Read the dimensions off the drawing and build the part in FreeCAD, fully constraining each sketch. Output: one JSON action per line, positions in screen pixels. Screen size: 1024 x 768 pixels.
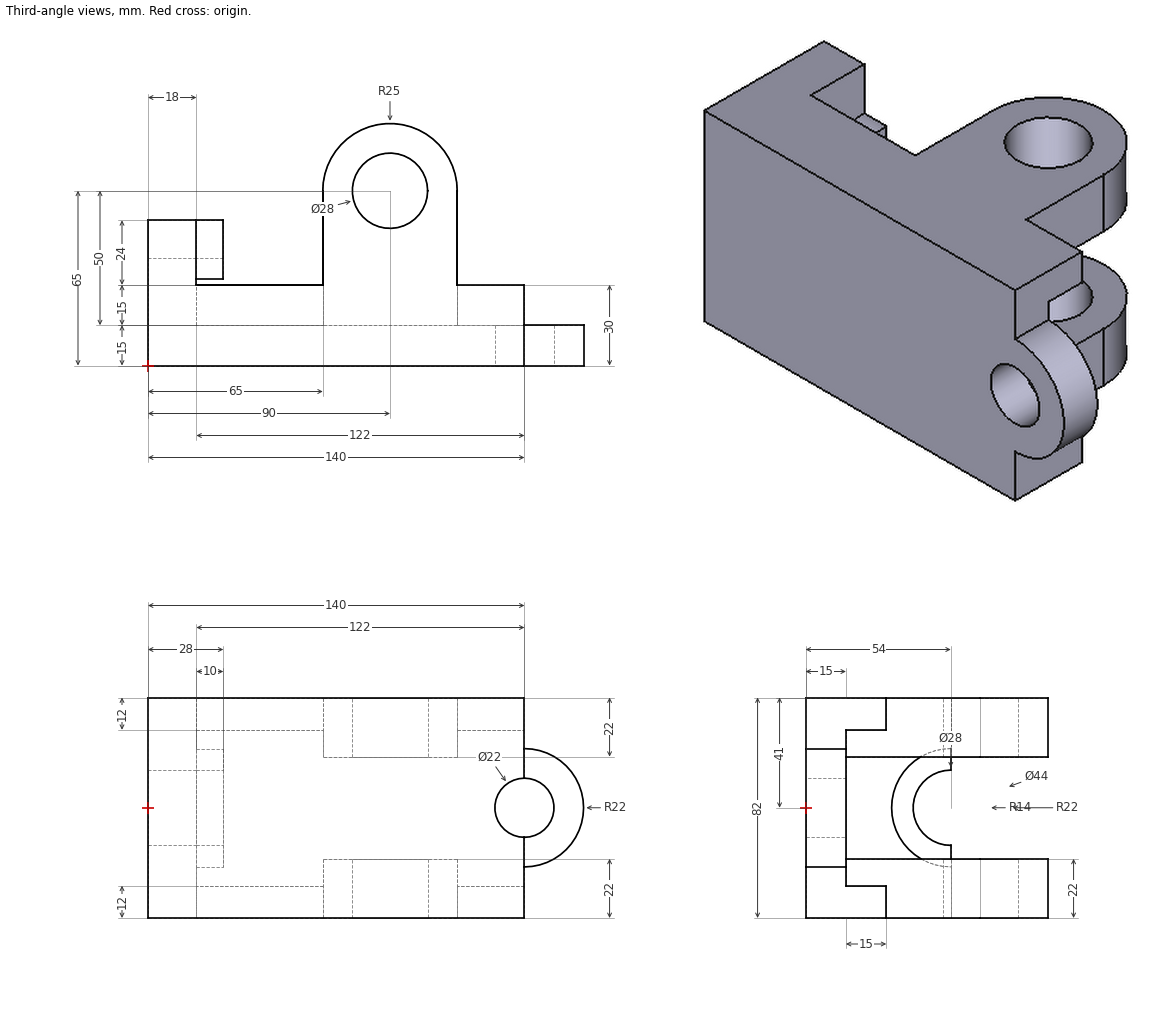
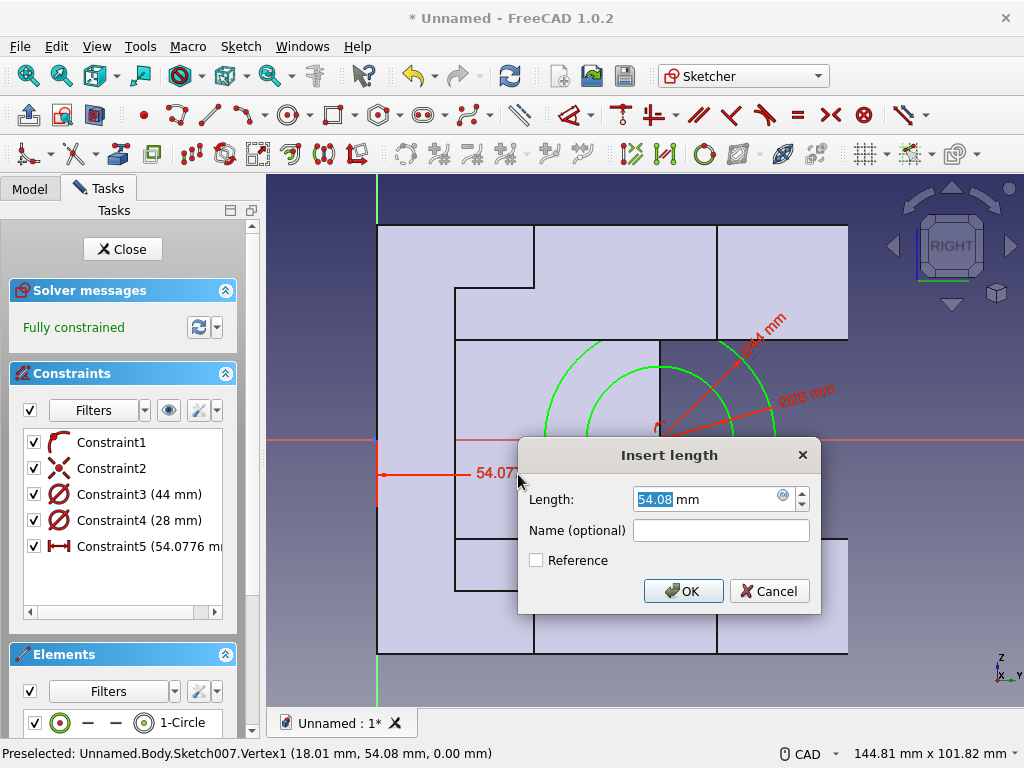
{"action": "type", "text": "54"}
{"action": "key", "text": "Return"}
{"action": "key", "text": "Escape"}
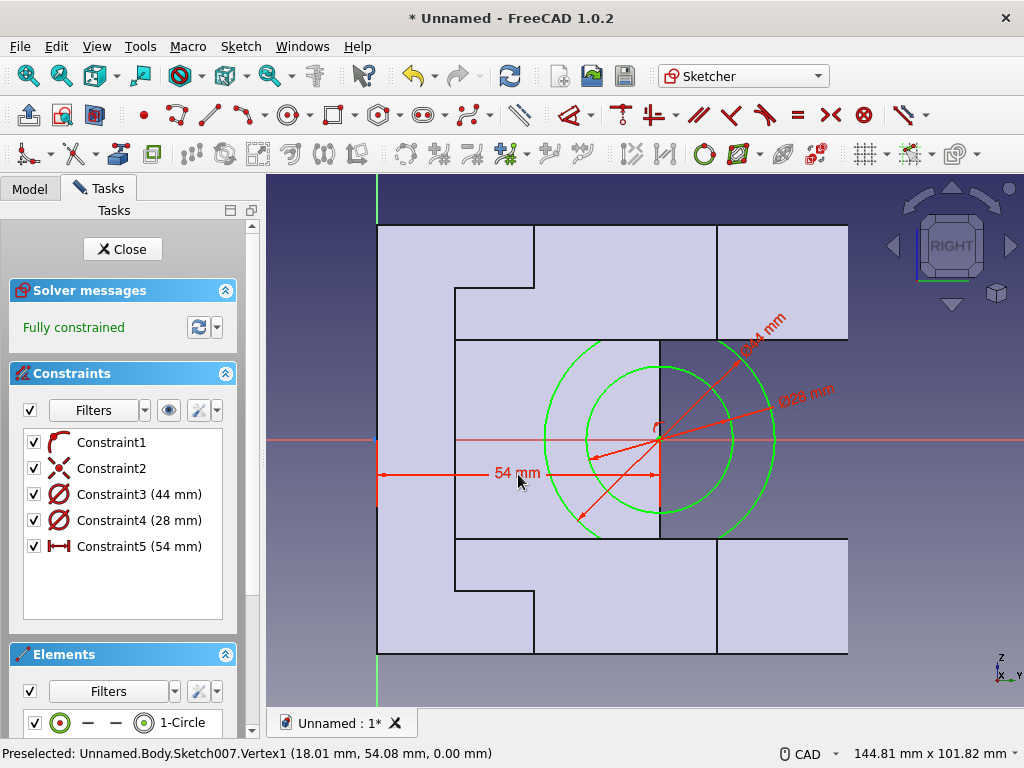
{"action": "left_click", "coordinate": [123, 249]}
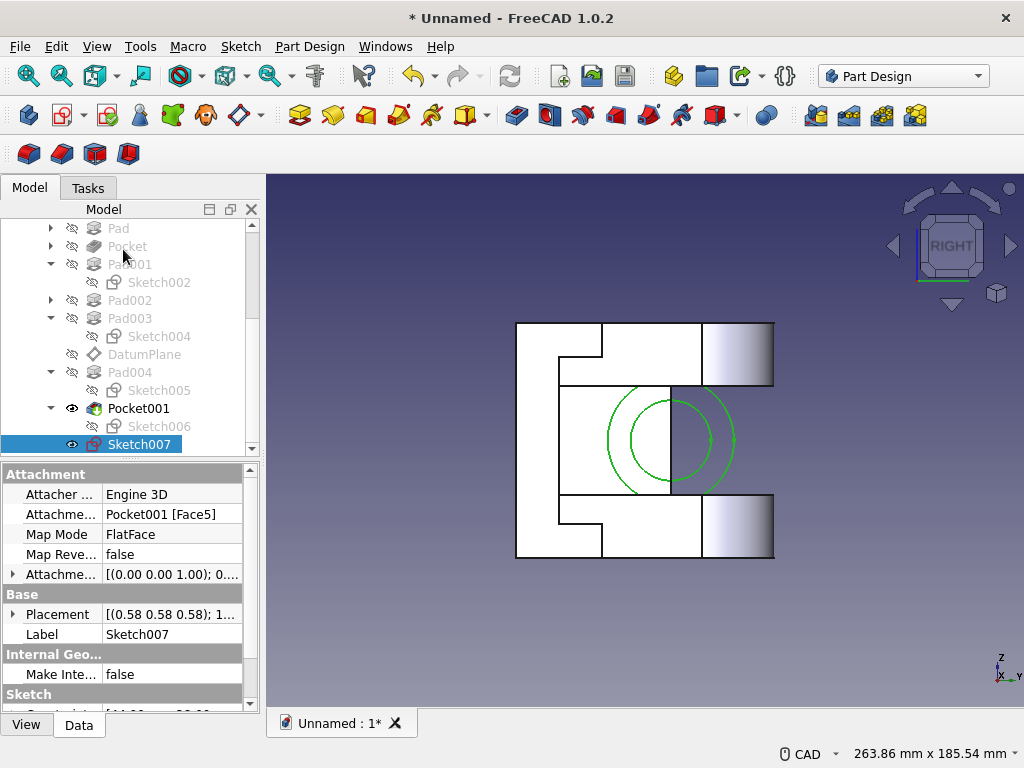
{"action": "left_click", "coordinate": [300, 116]}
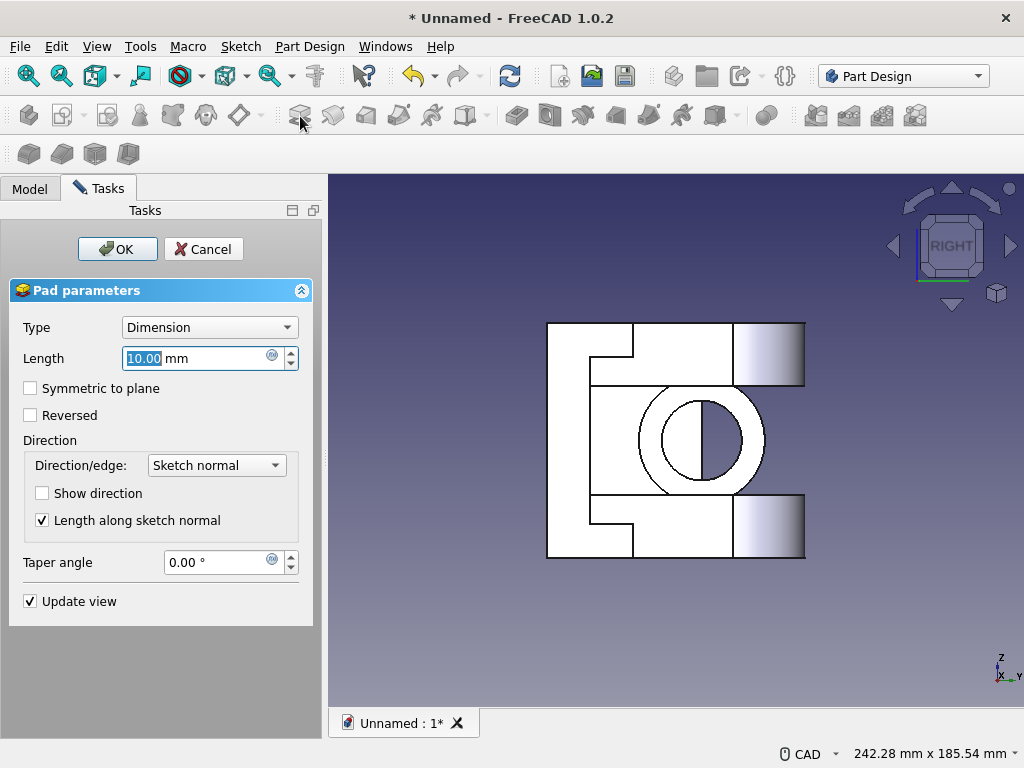
{"action": "type", "text": "10"}
{"action": "key", "text": "Tab"}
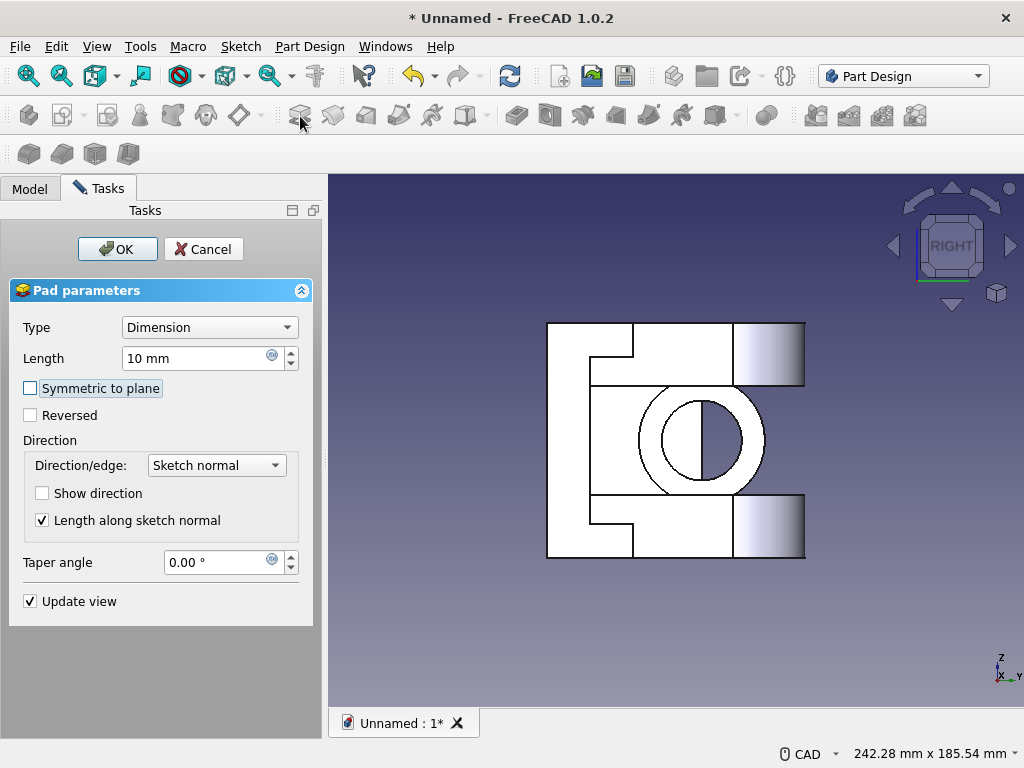
{"action": "left_click", "coordinate": [118, 249]}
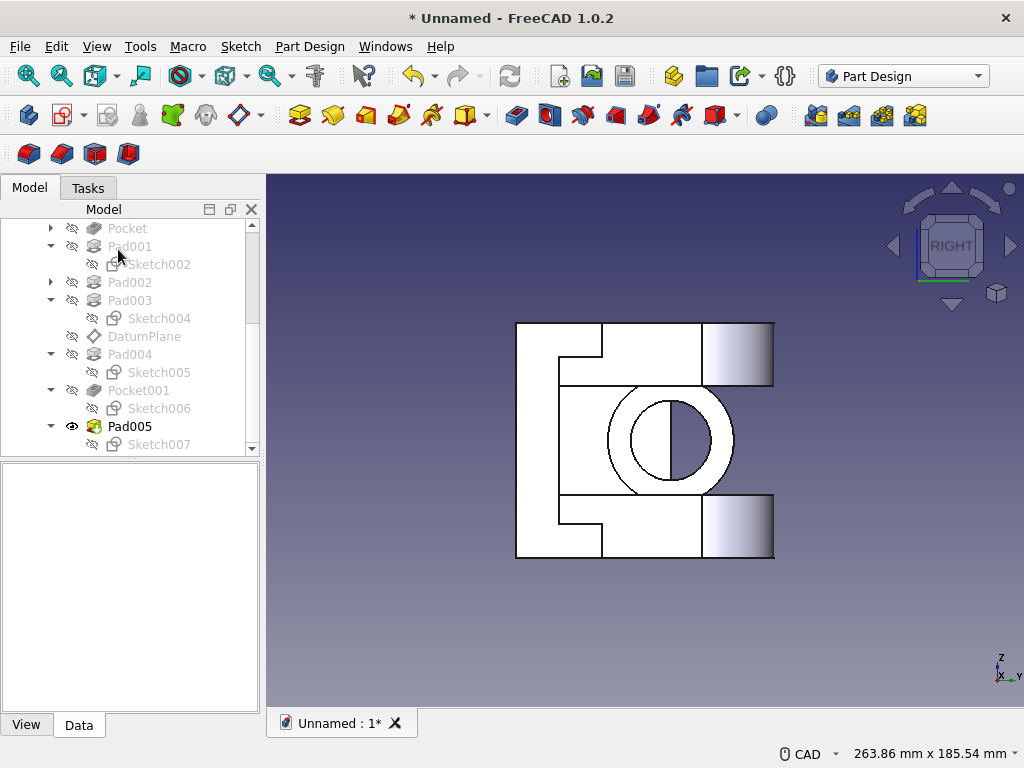
{"action": "key", "text": "v f"}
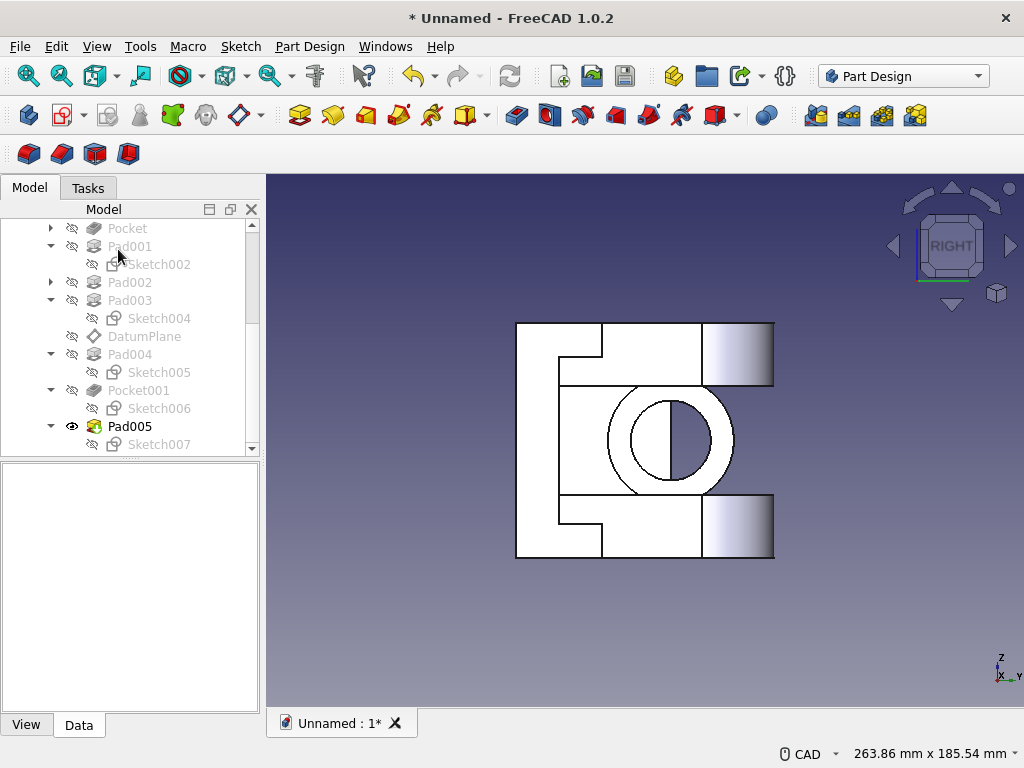
{"action": "left_click", "coordinate": [583, 406]}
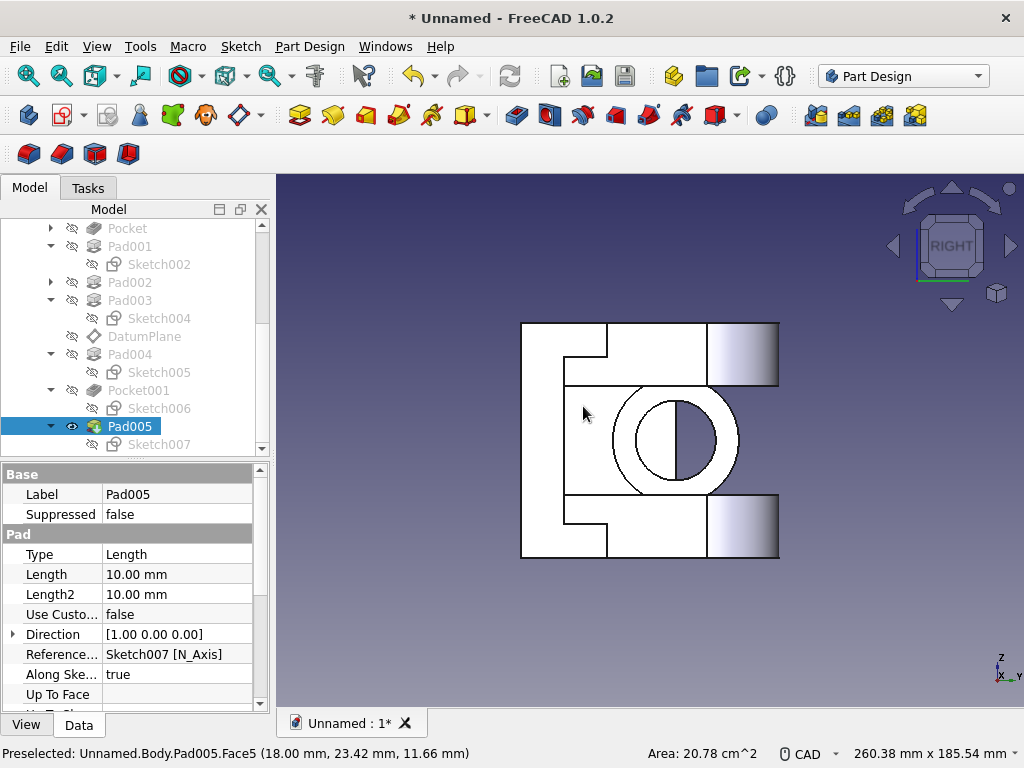
{"action": "left_click", "coordinate": [62, 116]}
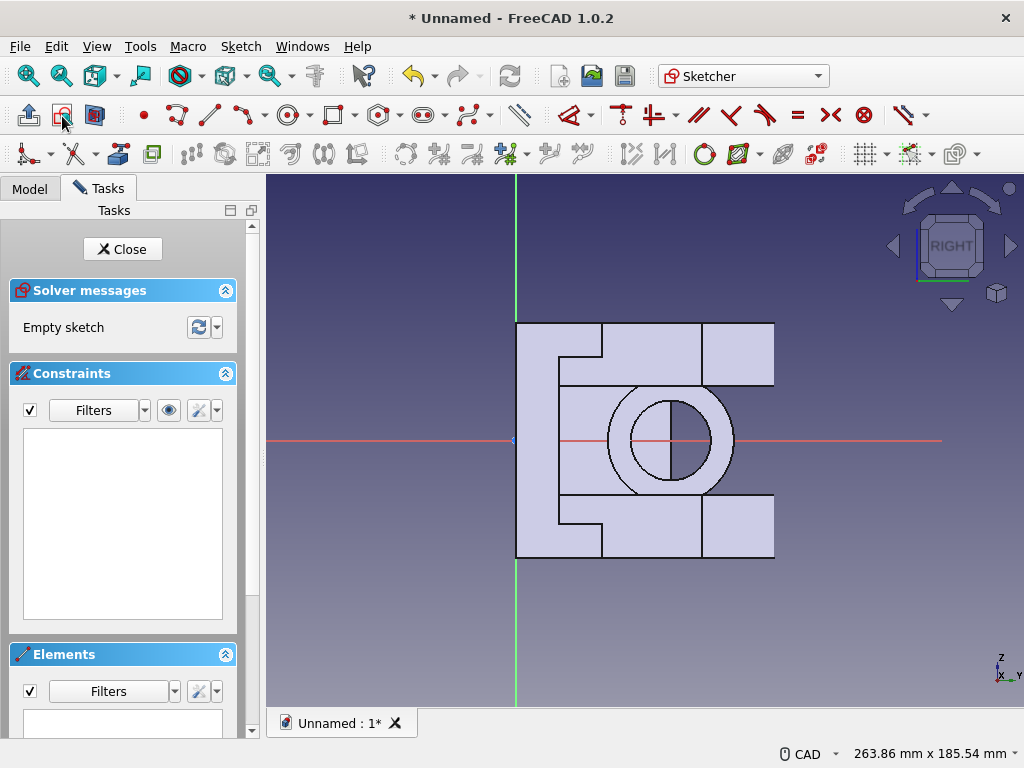
{"action": "scroll", "coordinate": [684, 441], "scroll_direction": "up", "scroll_amount": 3}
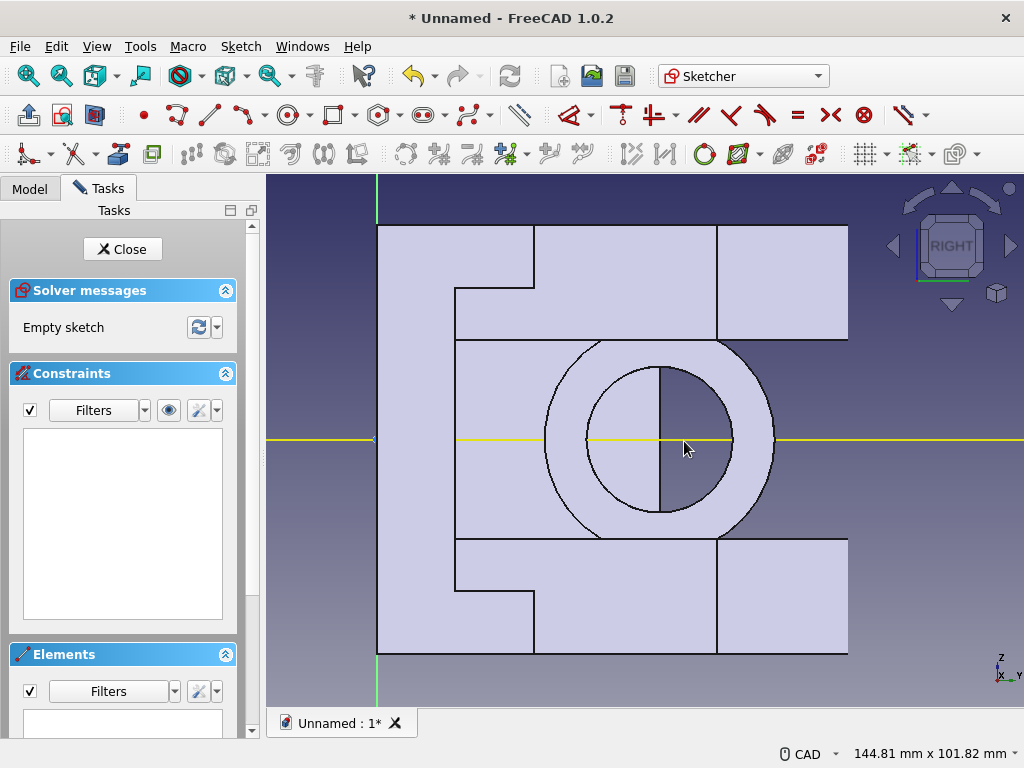
{"action": "key", "text": "g l"}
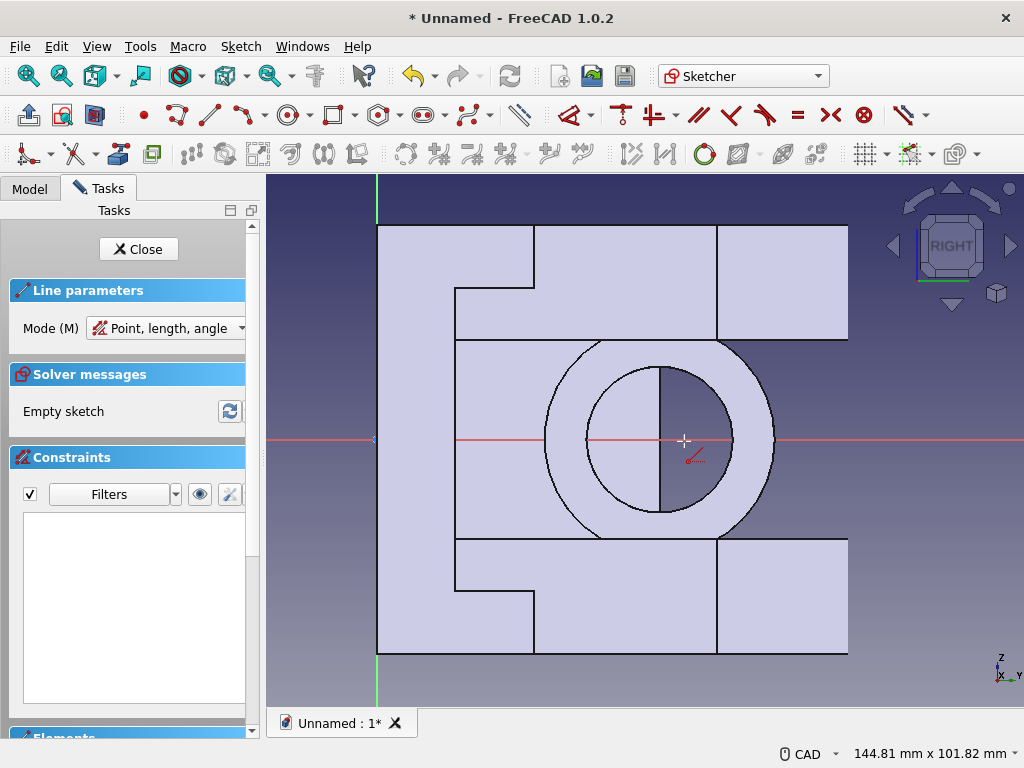
{"action": "left_click", "coordinate": [660, 325]}
{"action": "left_click", "coordinate": [660, 366]}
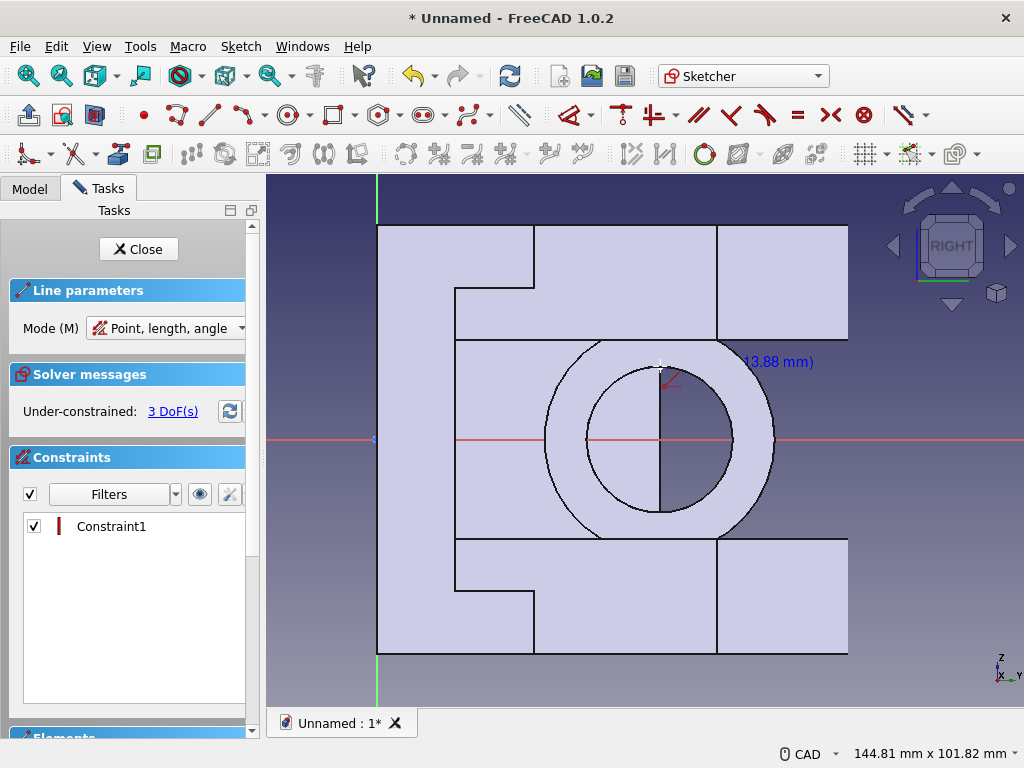
{"action": "left_click", "coordinate": [660, 513]}
{"action": "left_click", "coordinate": [660, 555]}